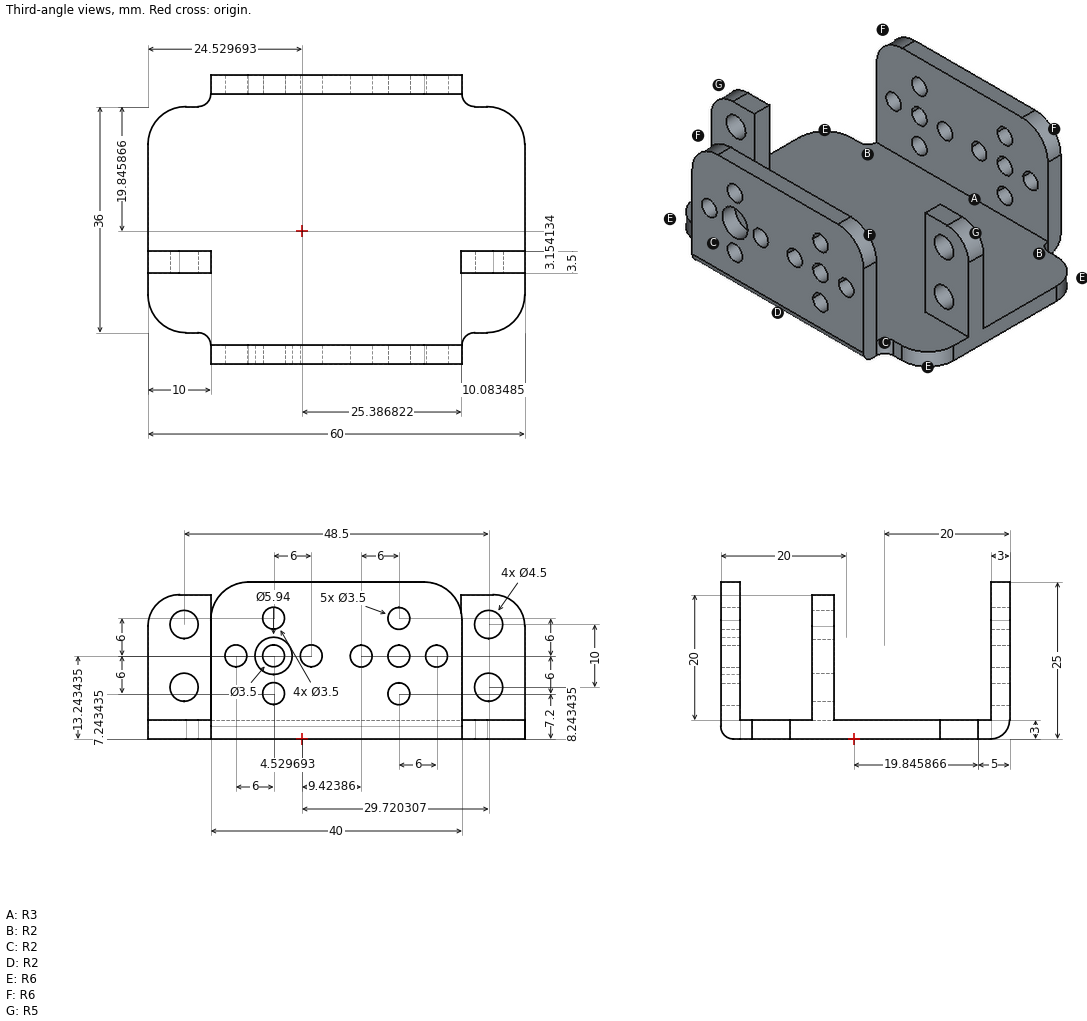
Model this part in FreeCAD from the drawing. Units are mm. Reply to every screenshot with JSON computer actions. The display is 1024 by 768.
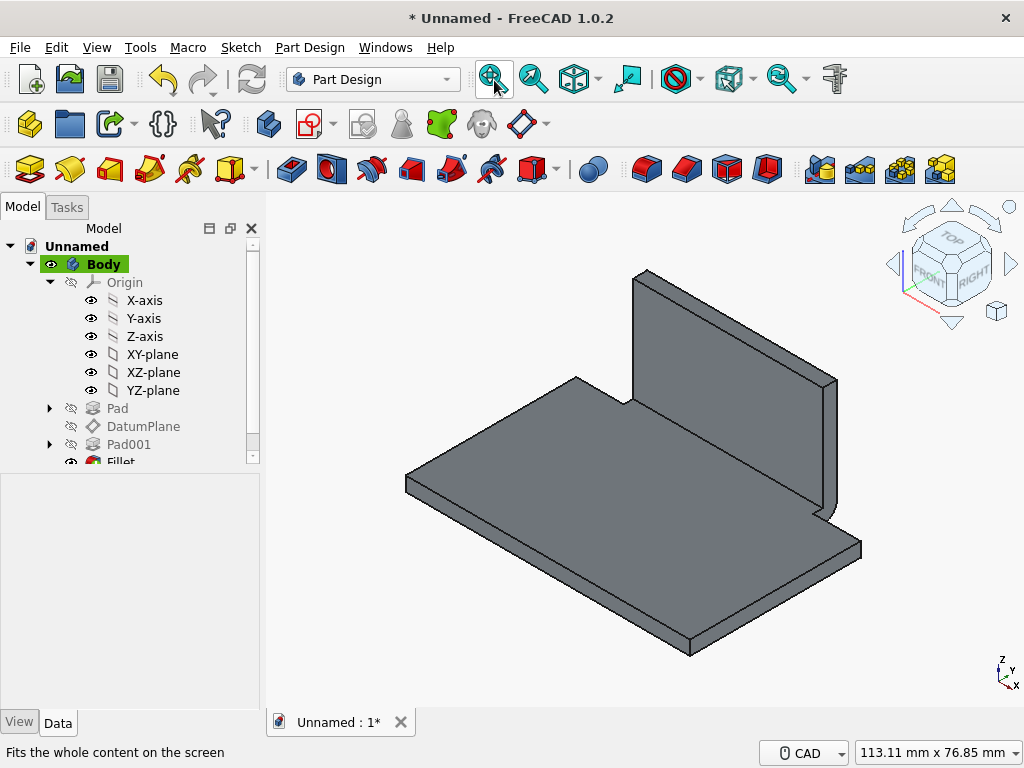
{"action": "key", "text": "2"}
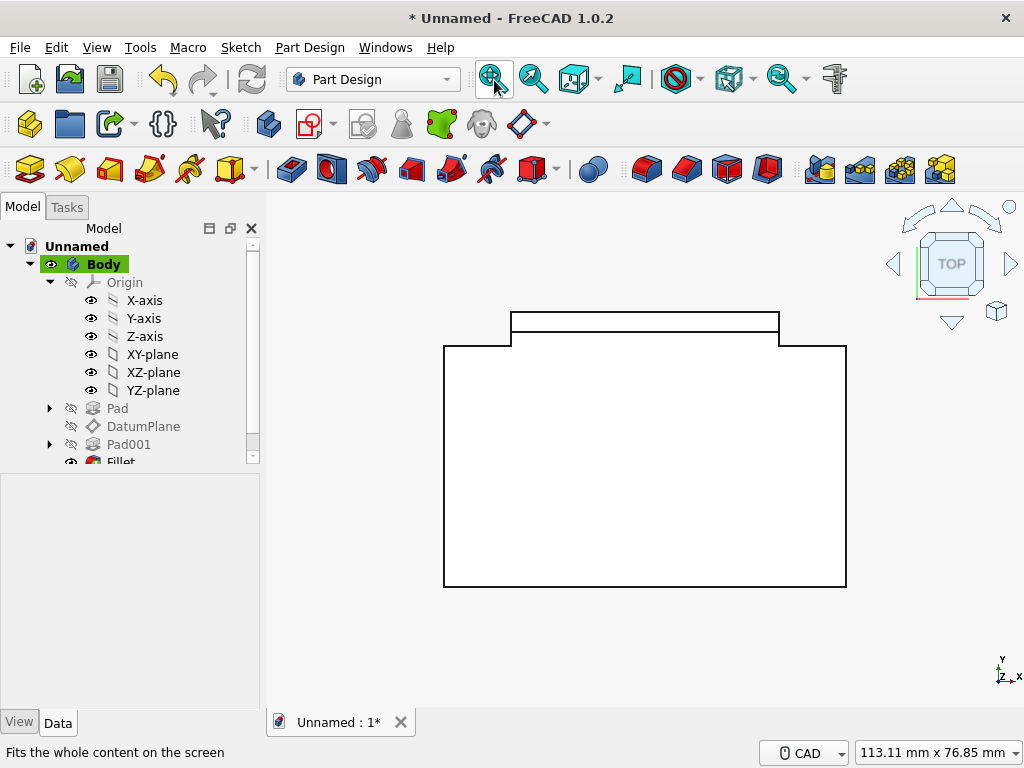
{"action": "scroll", "coordinate": [511, 345], "scroll_direction": "up", "scroll_amount": 4}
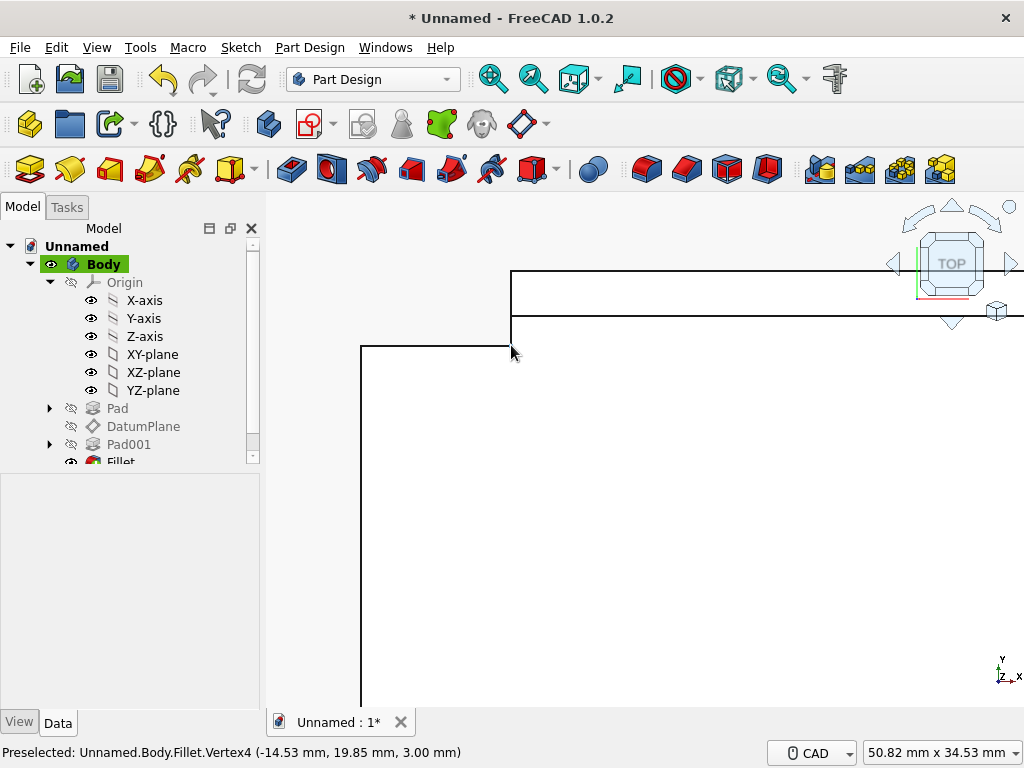
{"action": "left_click", "coordinate": [494, 80]}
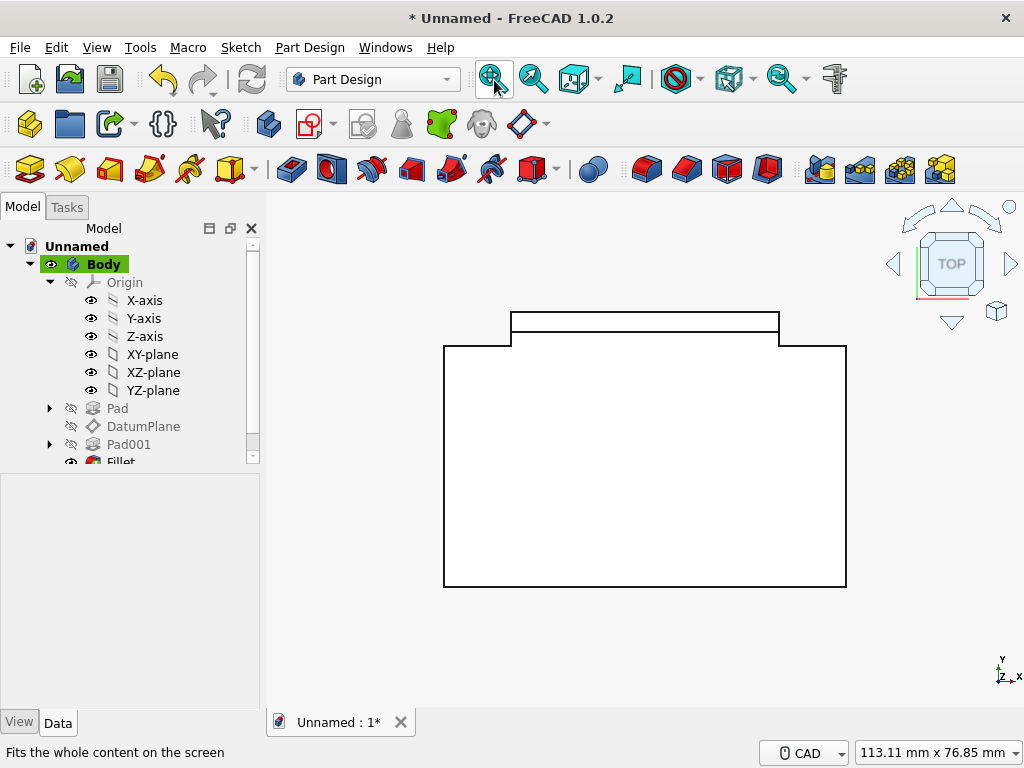
{"action": "key", "text": "1"}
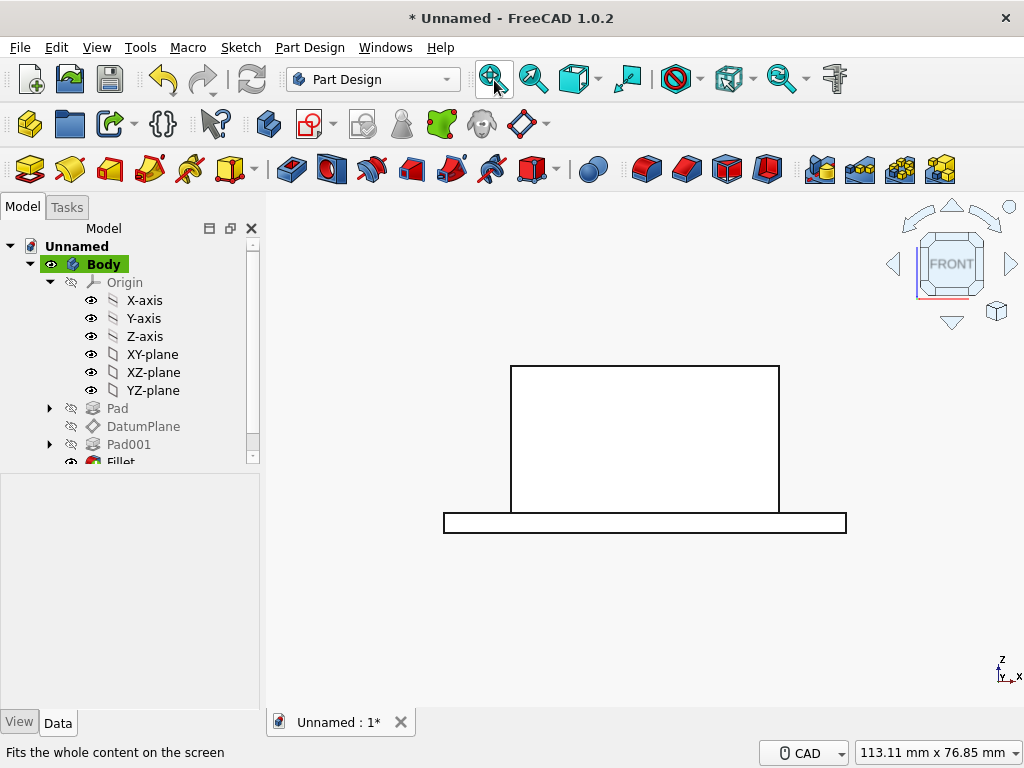
{"action": "scroll", "coordinate": [511, 522], "scroll_direction": "up", "scroll_amount": 4}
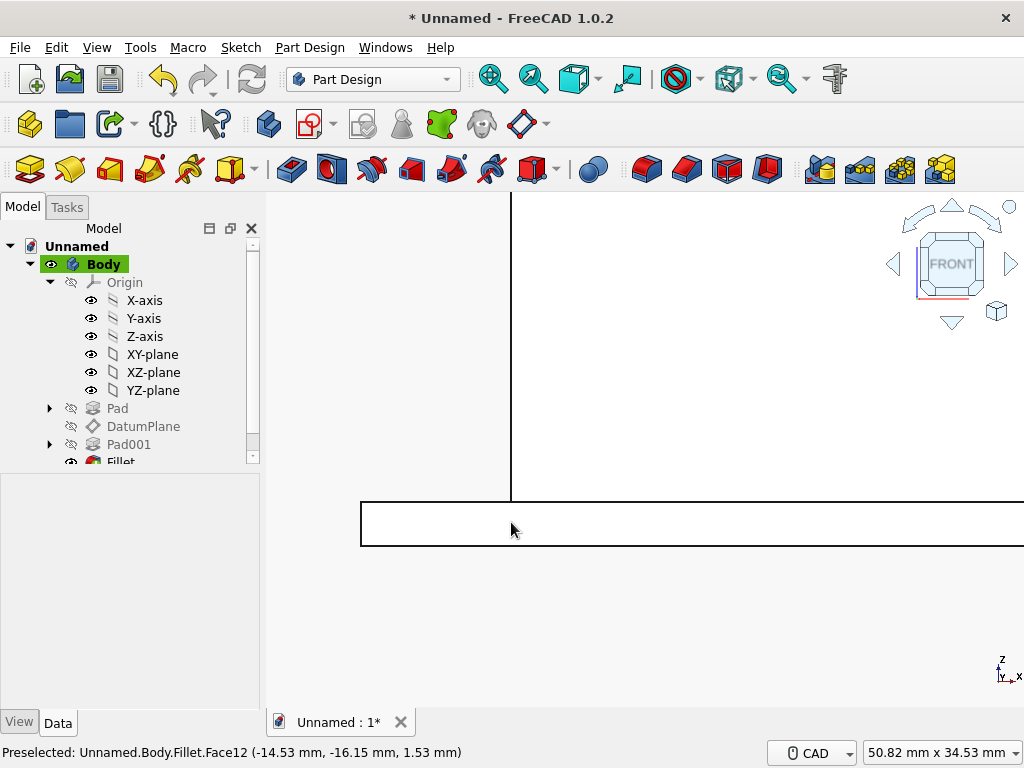
{"action": "left_click", "coordinate": [494, 80]}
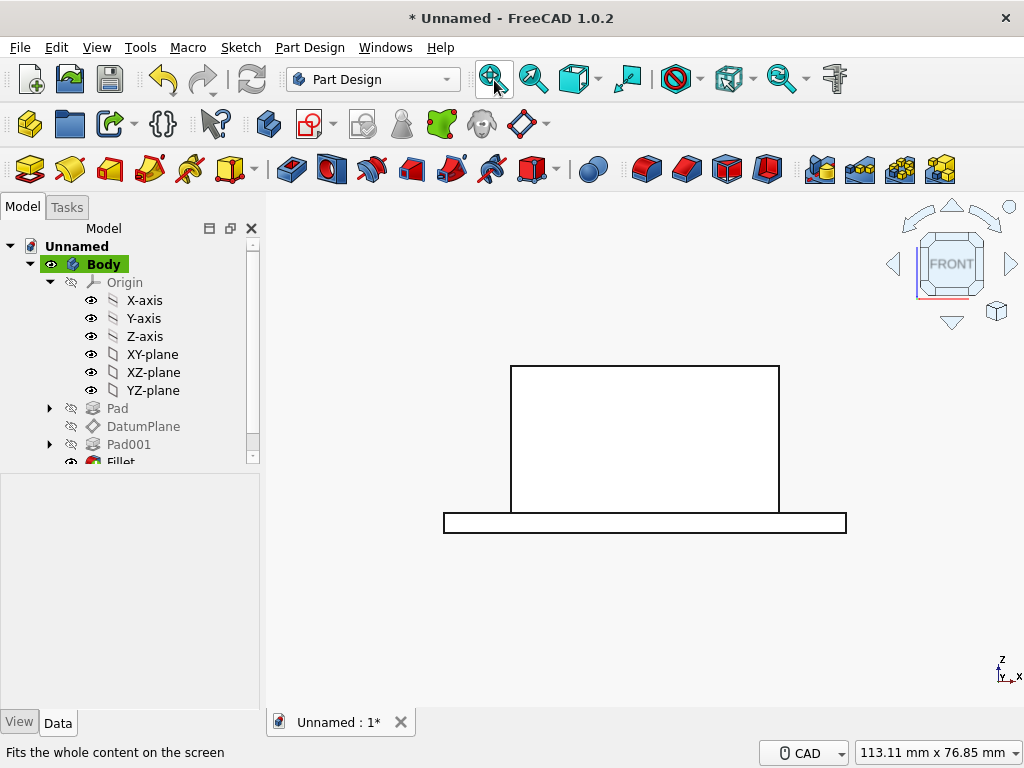
{"action": "key", "text": "3"}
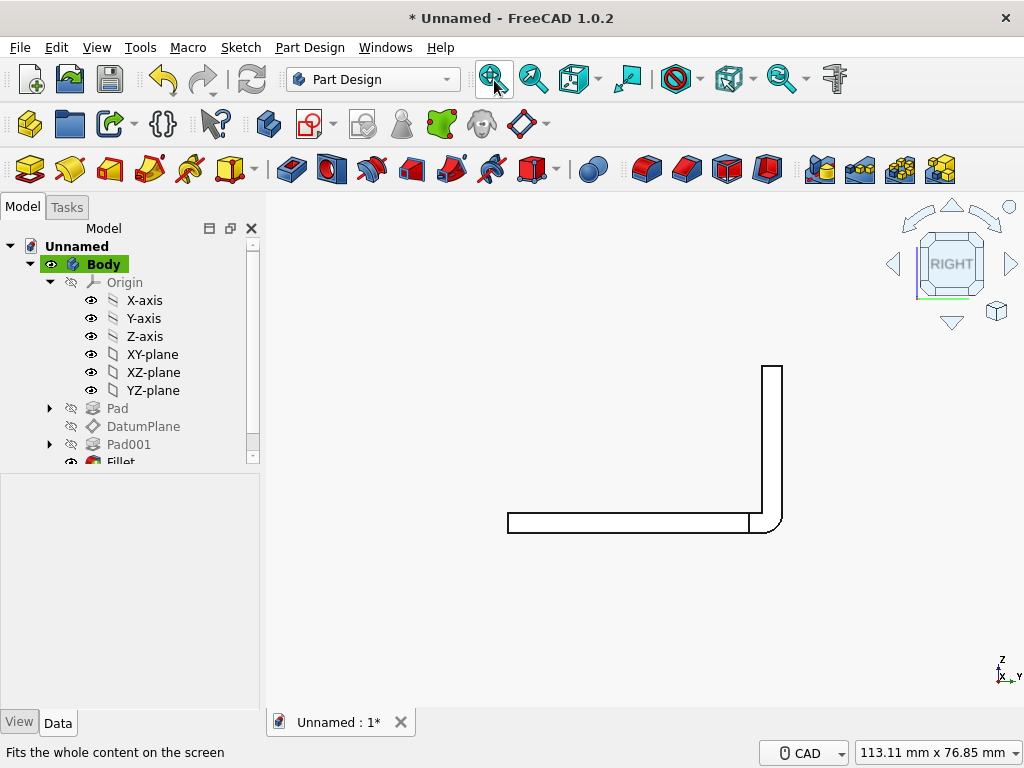
{"action": "left_click", "coordinate": [494, 80]}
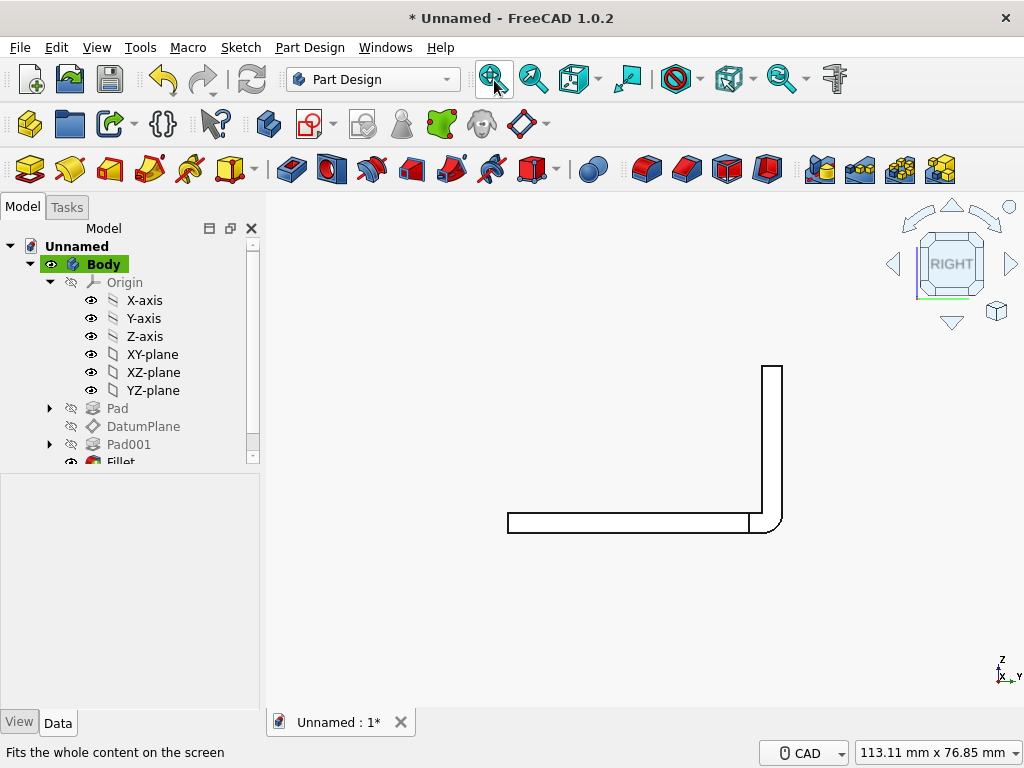
{"action": "scroll", "coordinate": [749, 522], "scroll_direction": "up", "scroll_amount": 4}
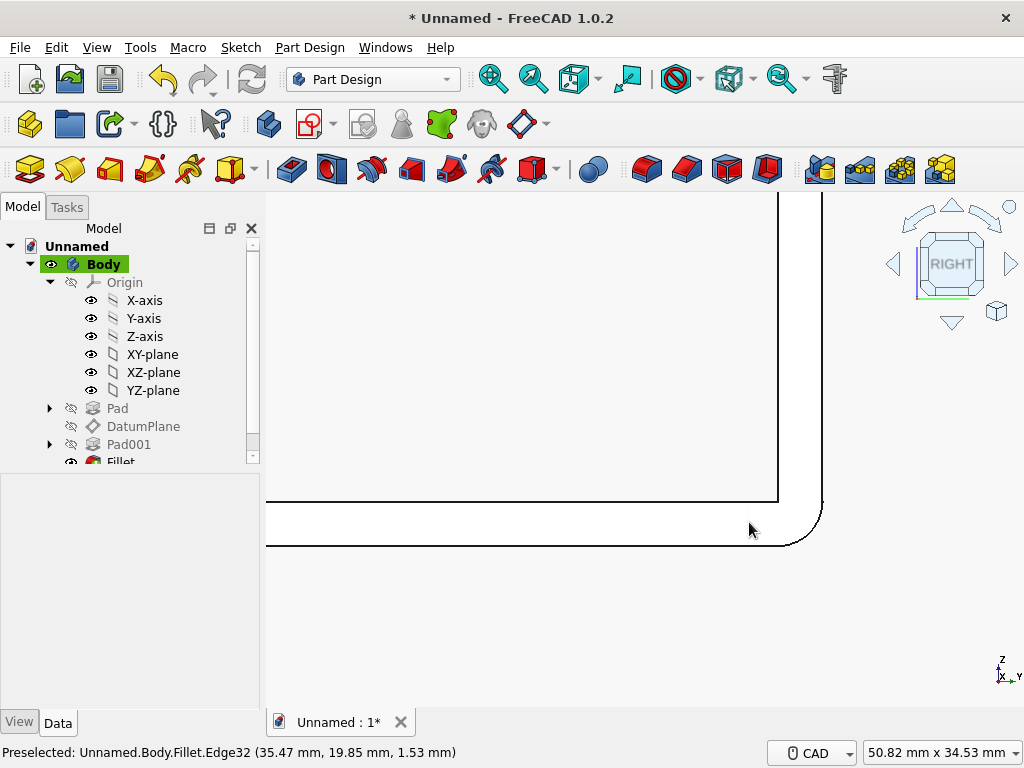
{"action": "left_click", "coordinate": [494, 80]}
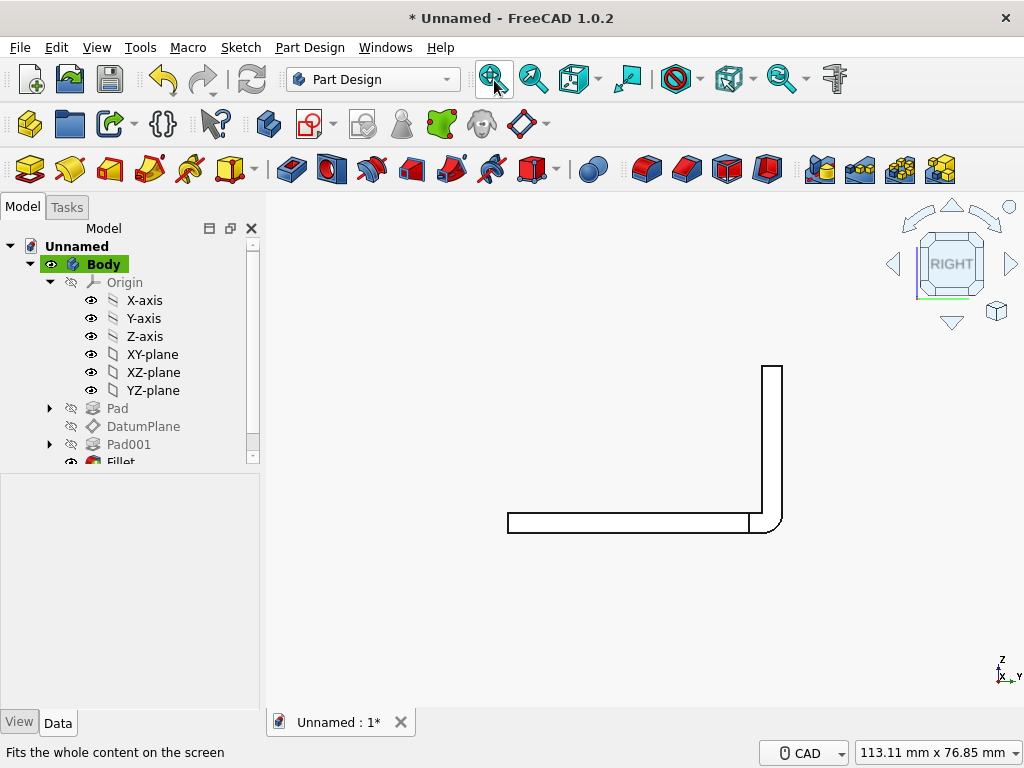
{"action": "key", "text": "5"}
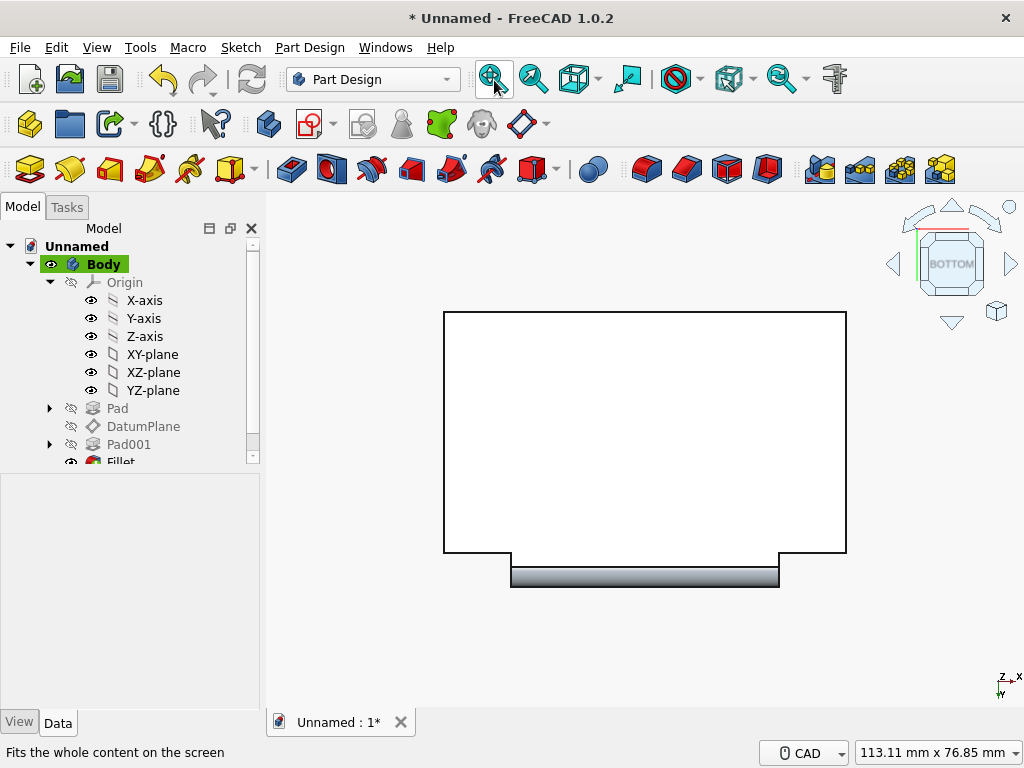
{"action": "scroll", "coordinate": [511, 552], "scroll_direction": "up", "scroll_amount": 4}